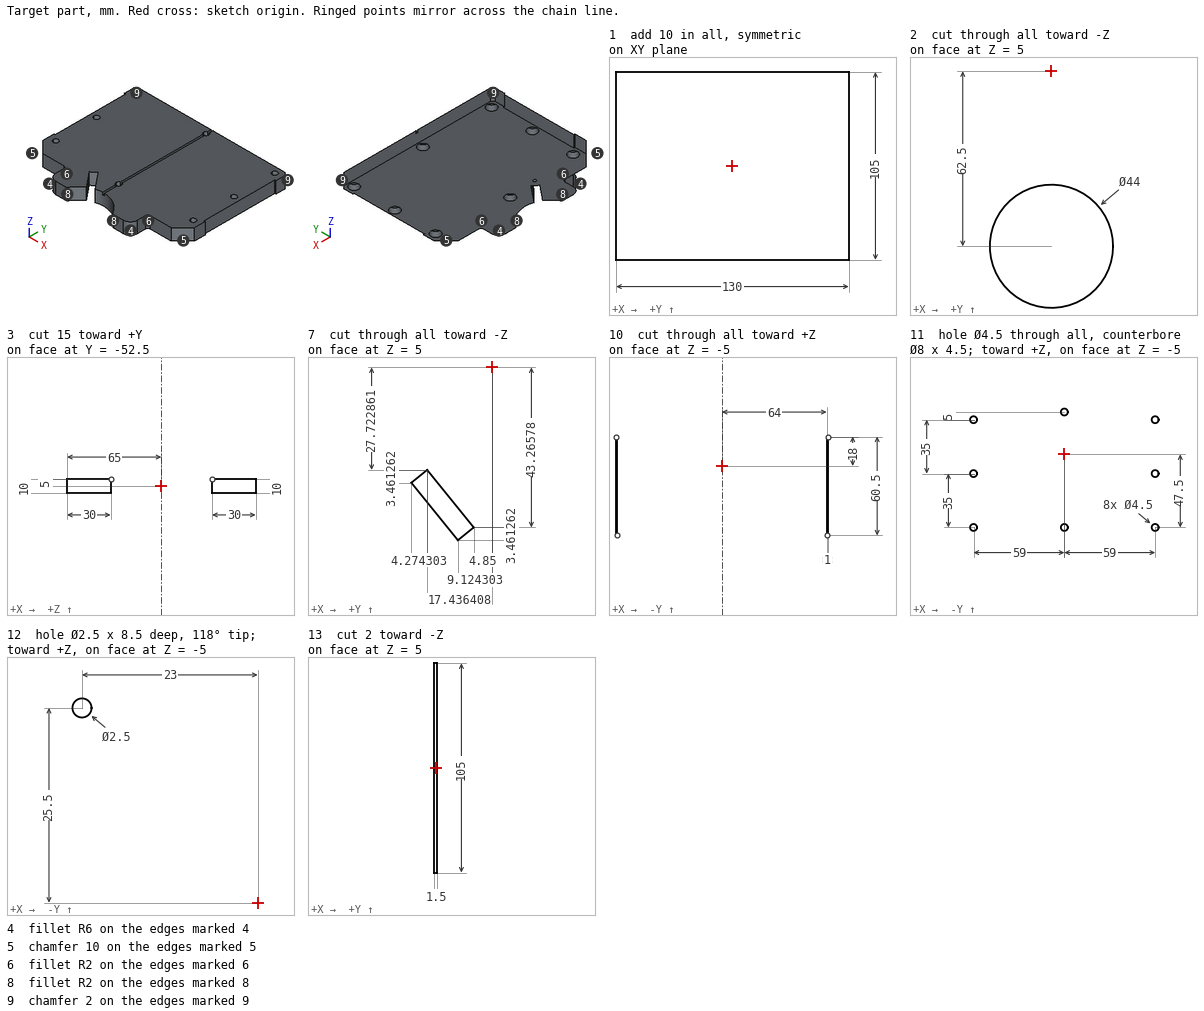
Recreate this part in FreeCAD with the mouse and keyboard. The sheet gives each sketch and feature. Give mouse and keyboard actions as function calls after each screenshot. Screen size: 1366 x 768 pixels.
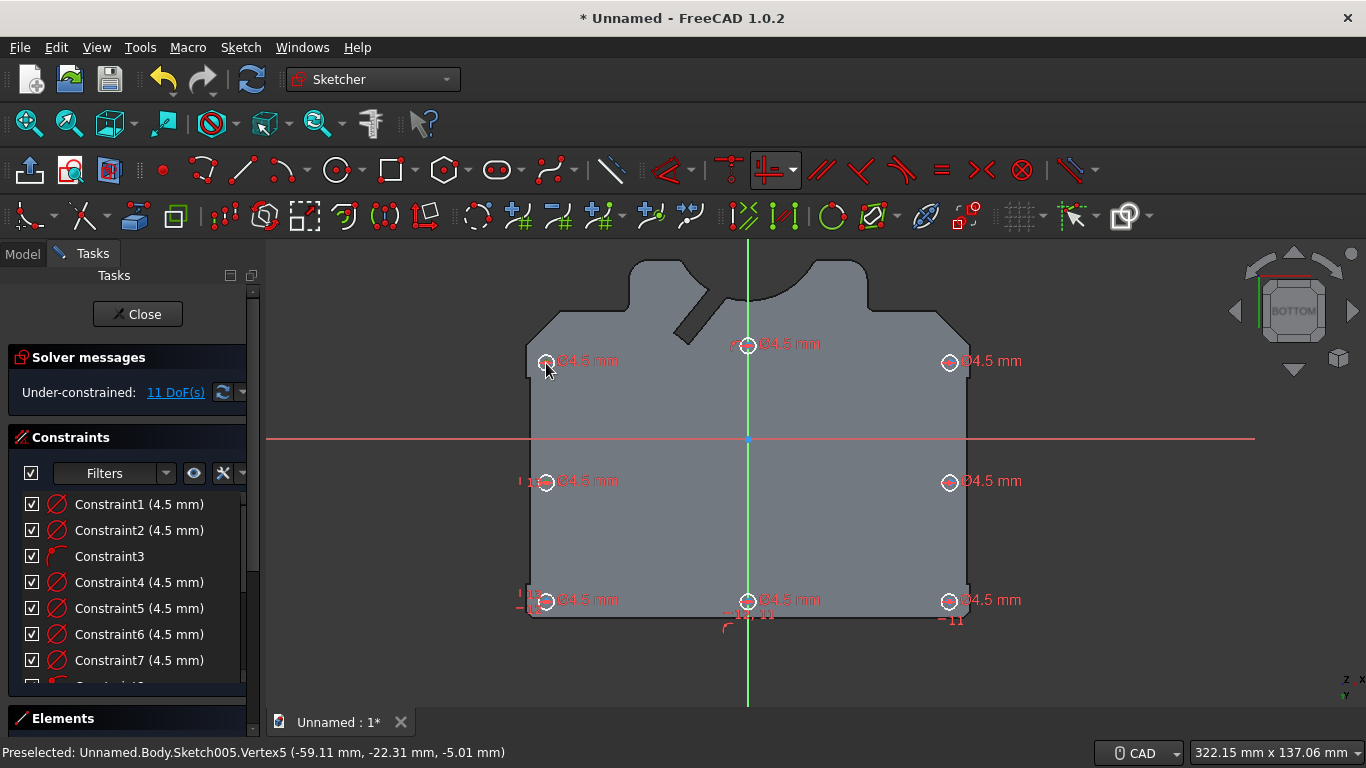
key(v)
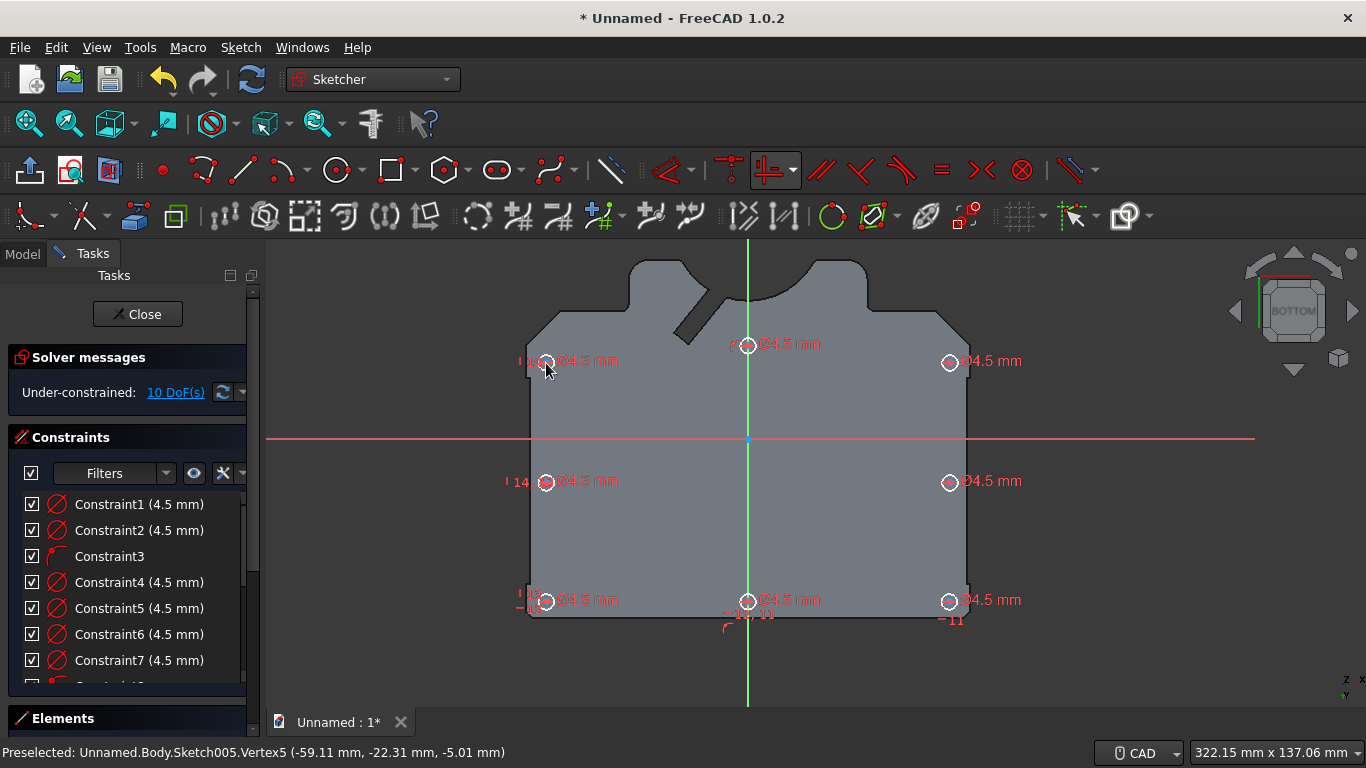
click(949, 602)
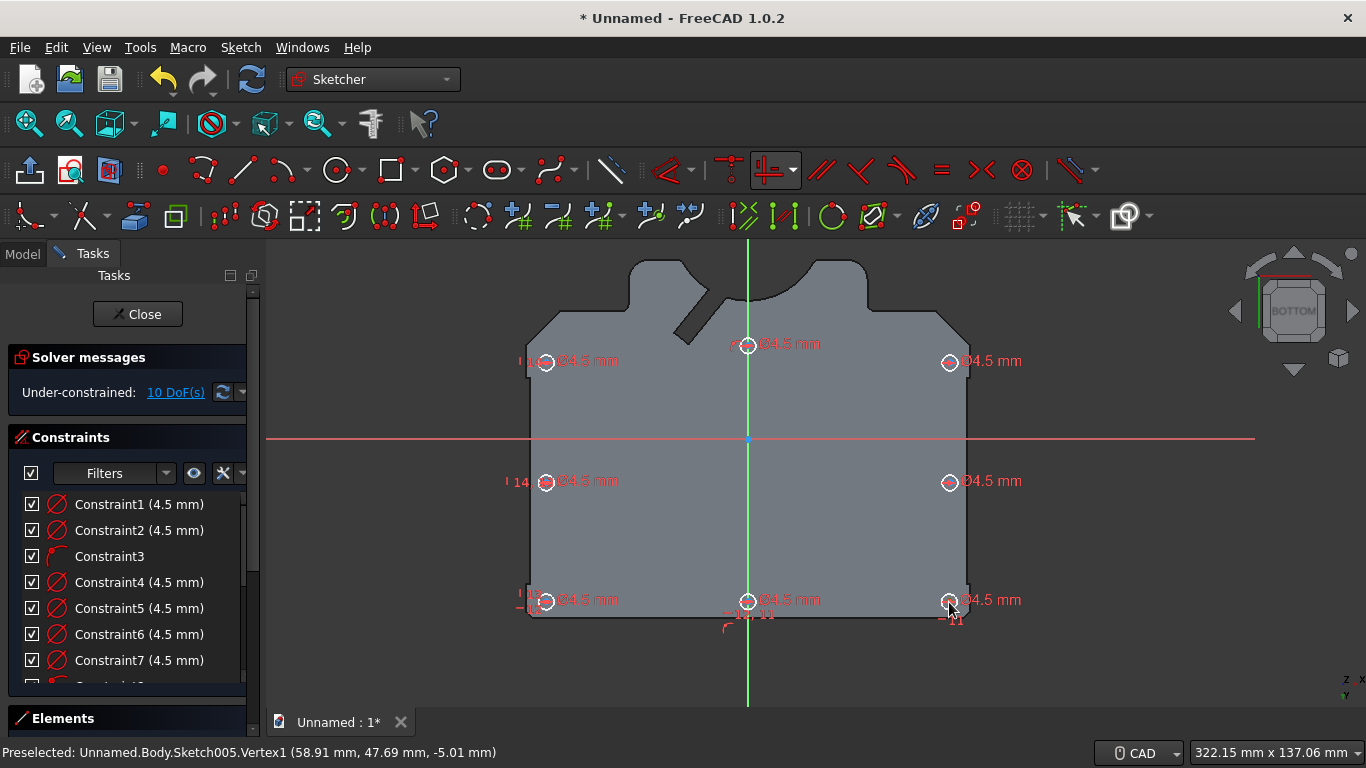
click(950, 363)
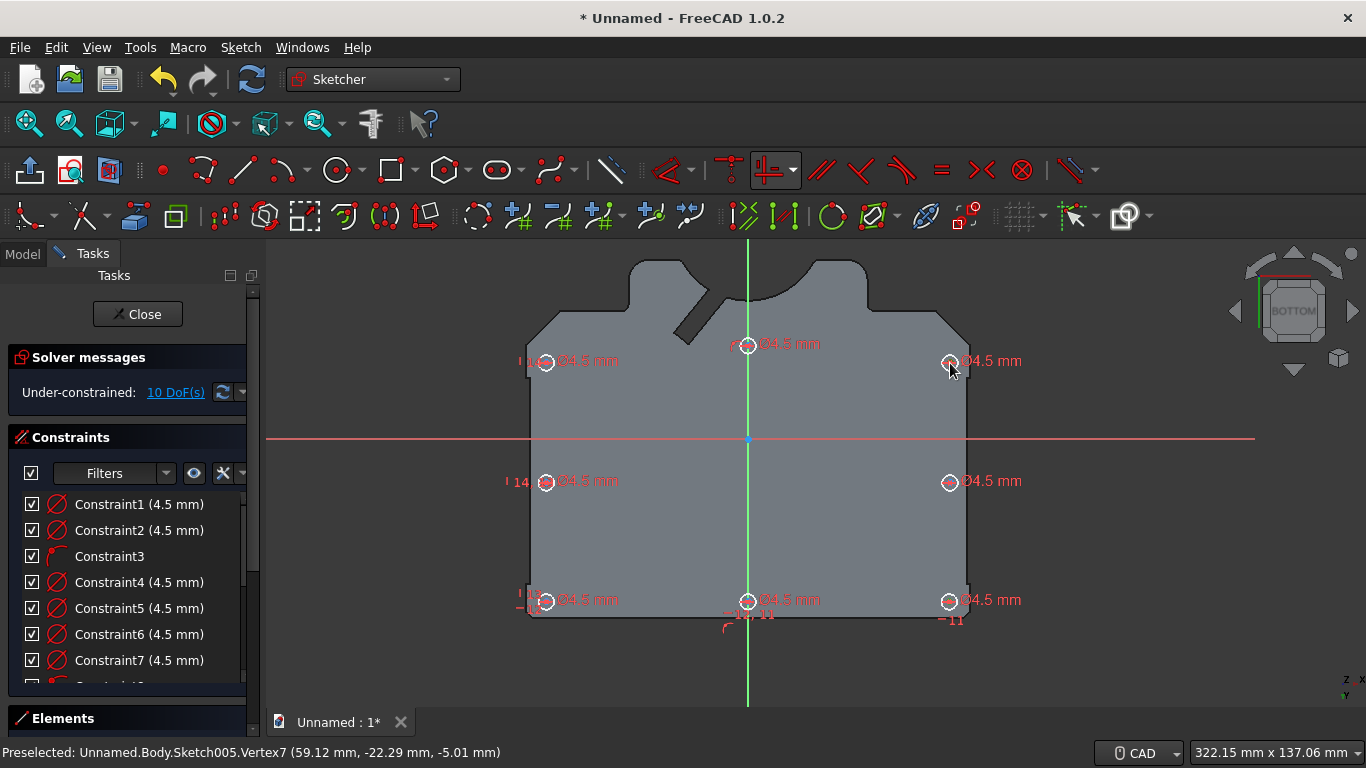
click(796, 170)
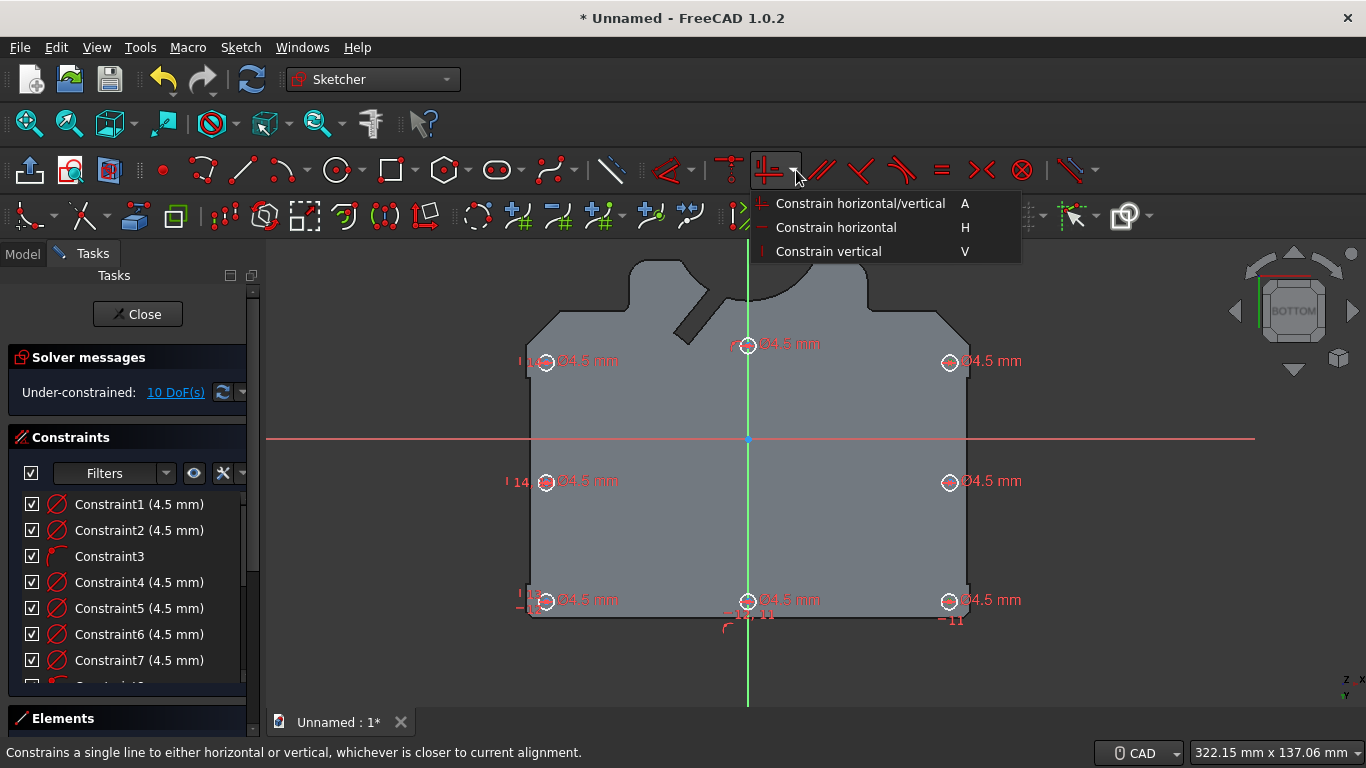
click(886, 251)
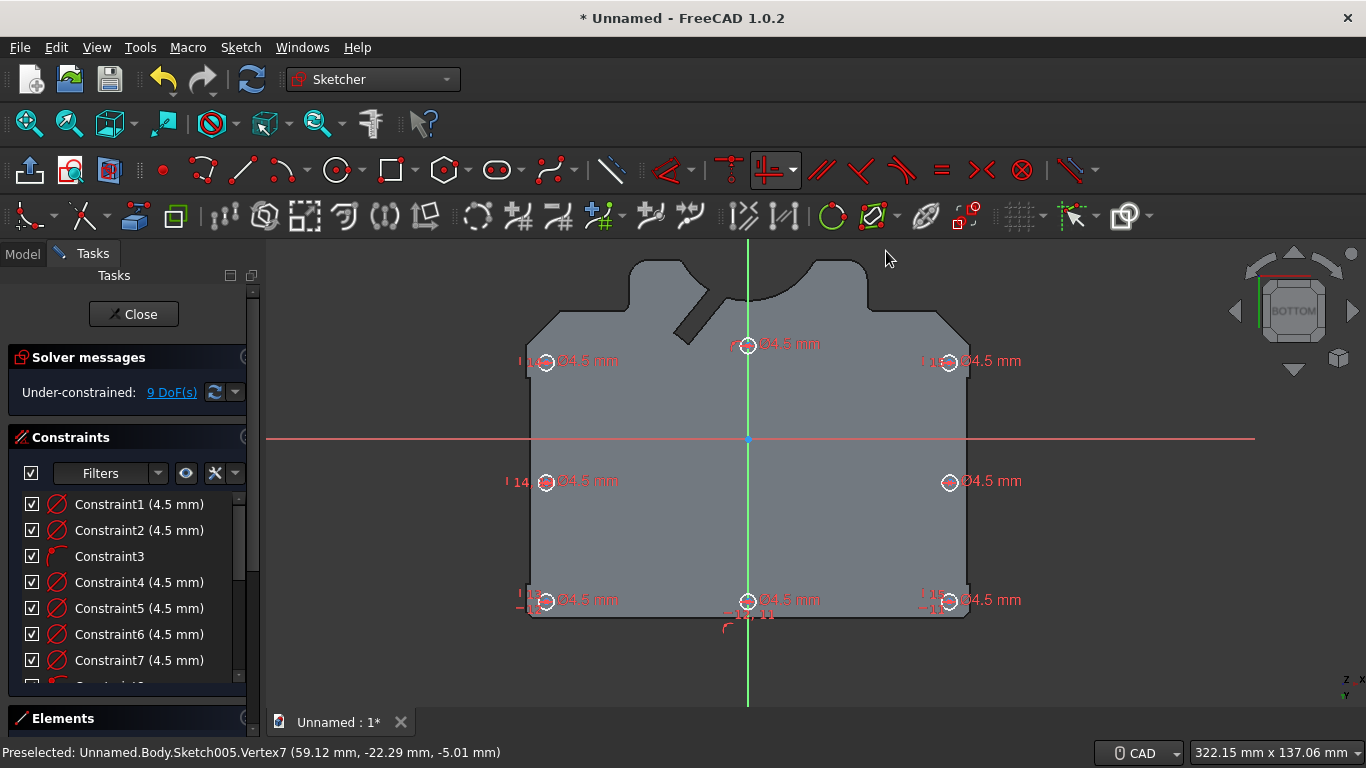
click(546, 363)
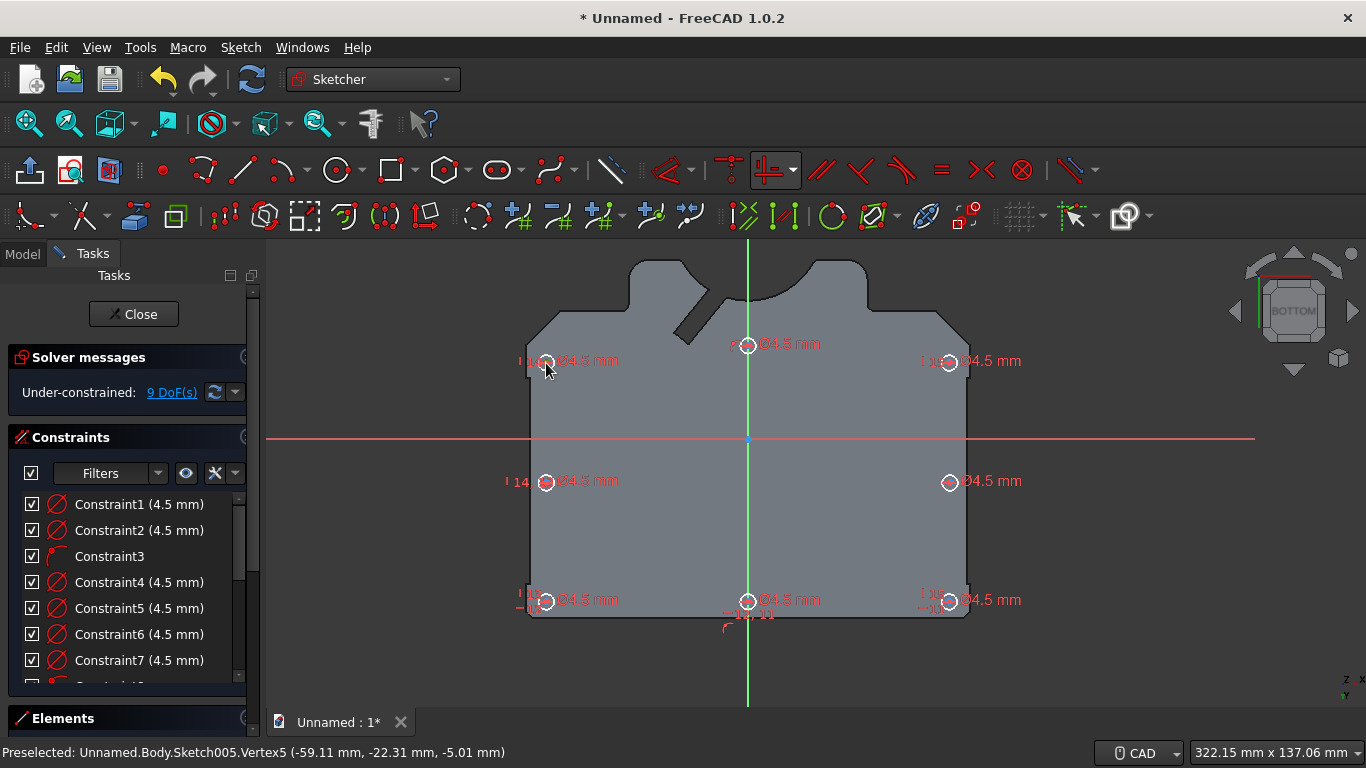
click(949, 363)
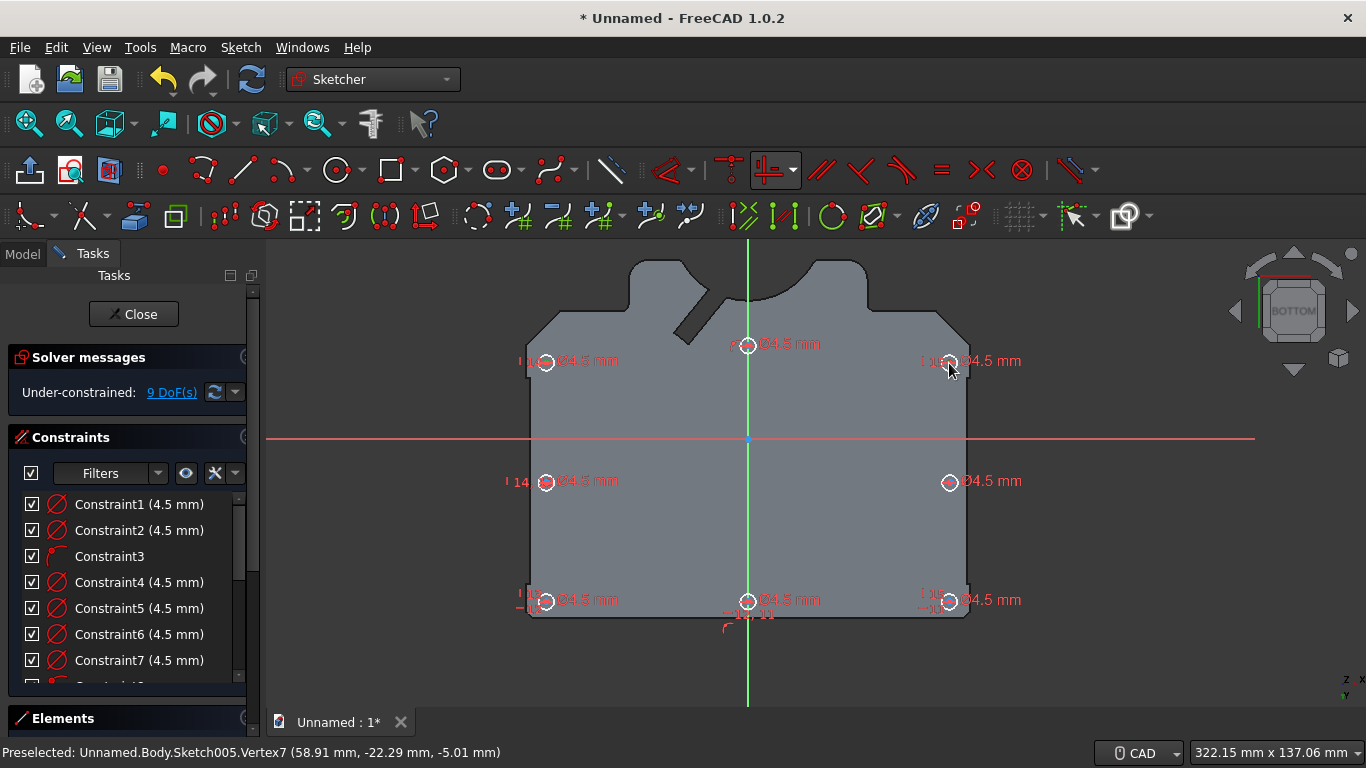
click(796, 170)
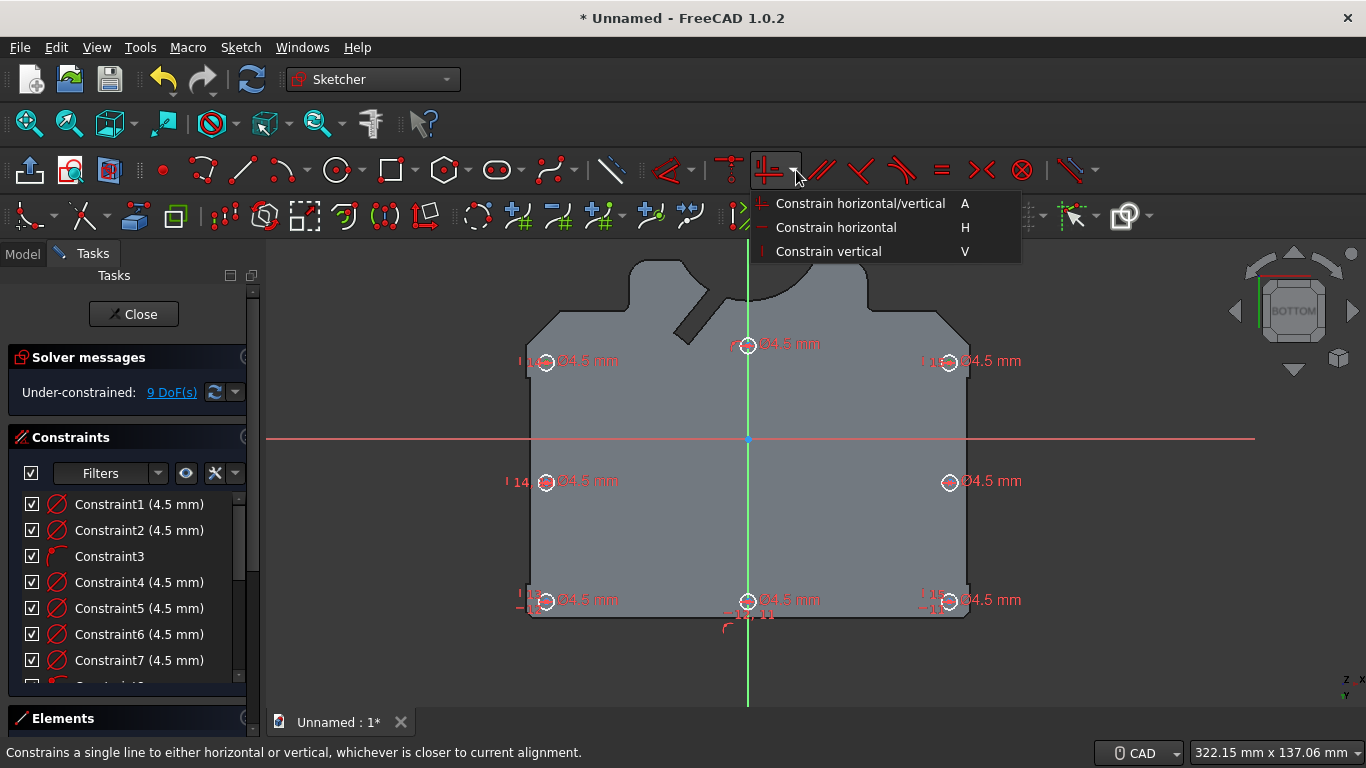
click(886, 227)